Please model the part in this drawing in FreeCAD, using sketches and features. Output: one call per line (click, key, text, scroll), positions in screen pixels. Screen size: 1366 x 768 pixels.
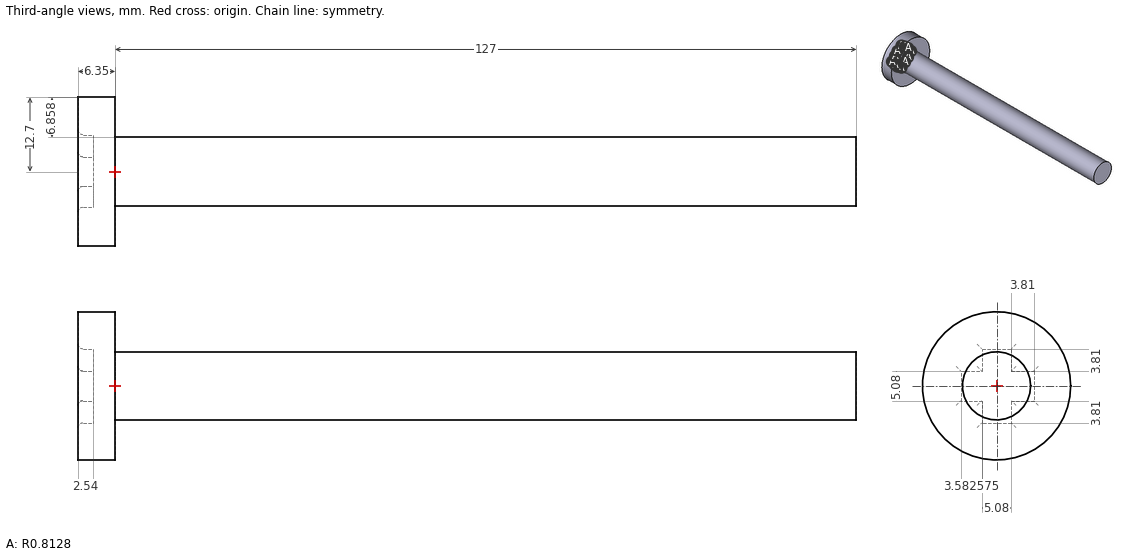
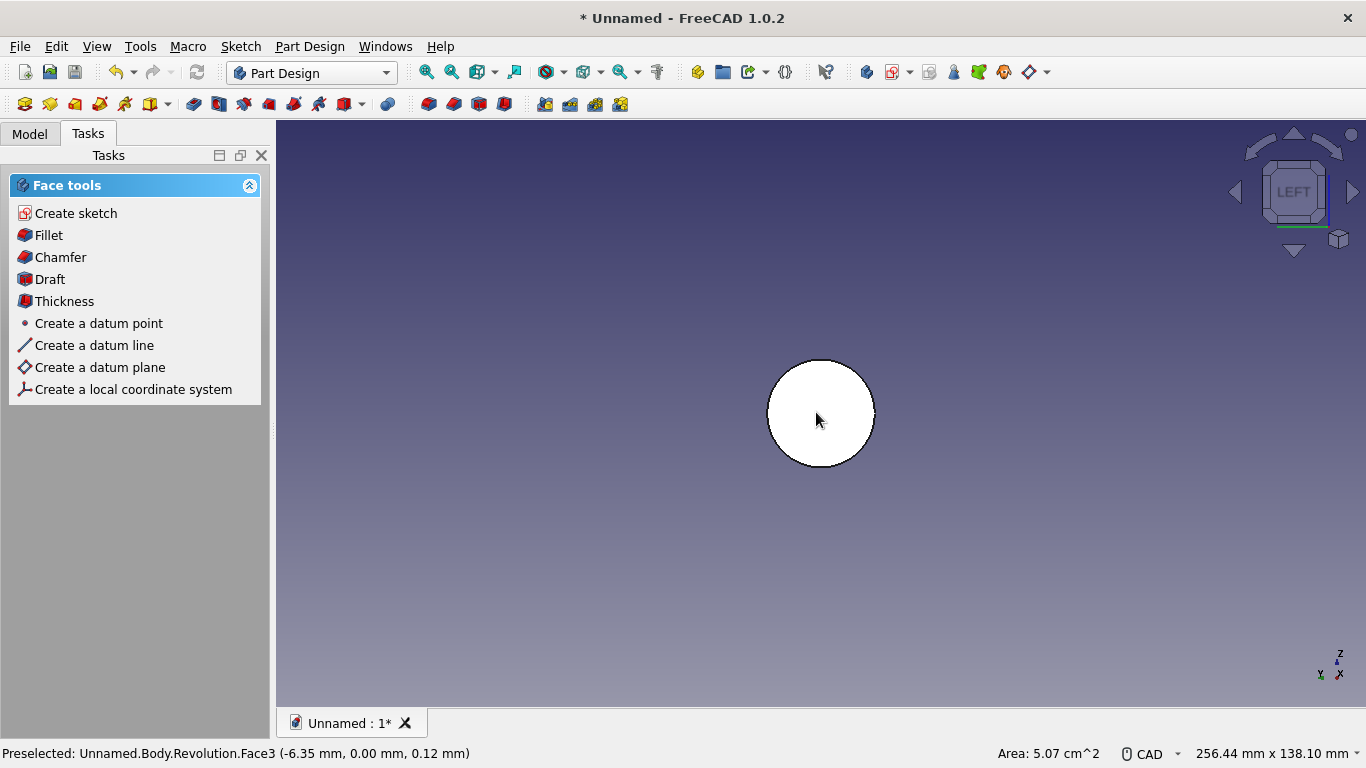
click(892, 72)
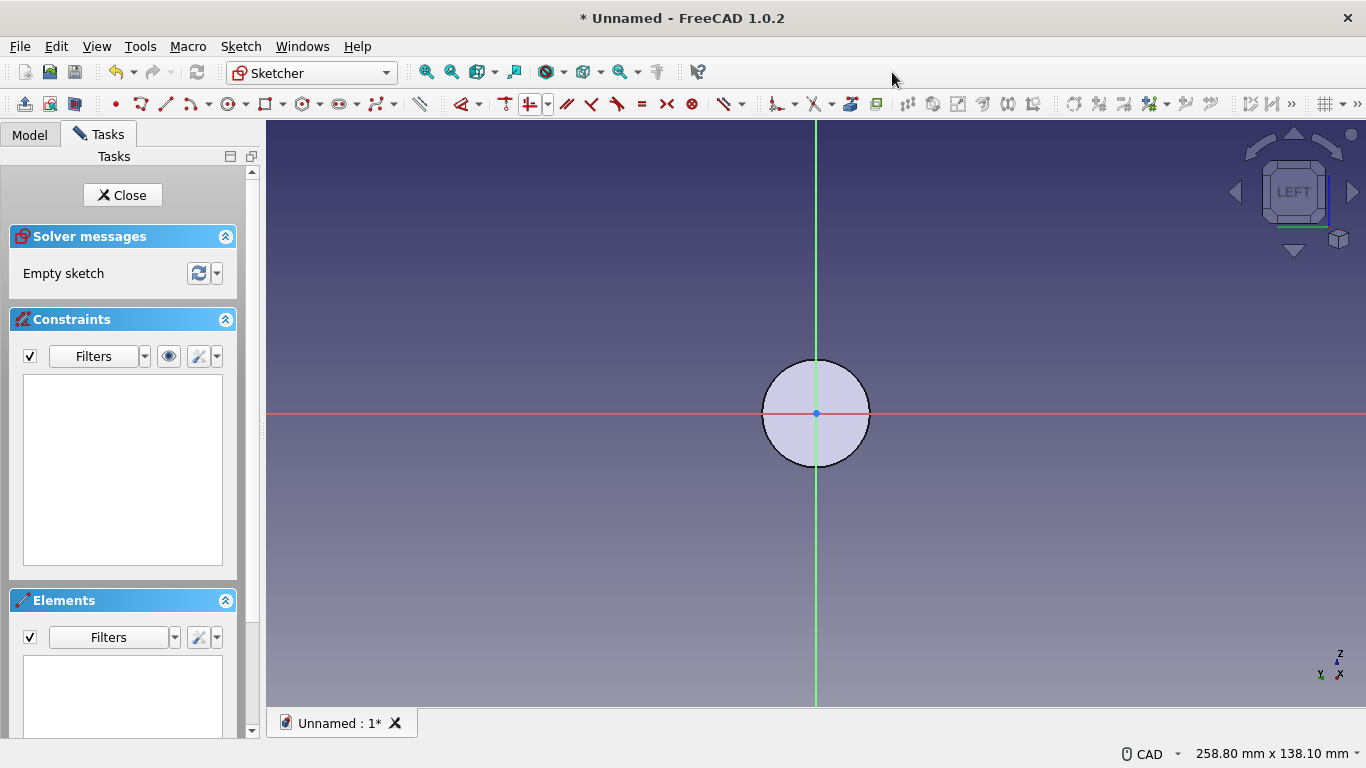
scroll(826, 414, up, 10)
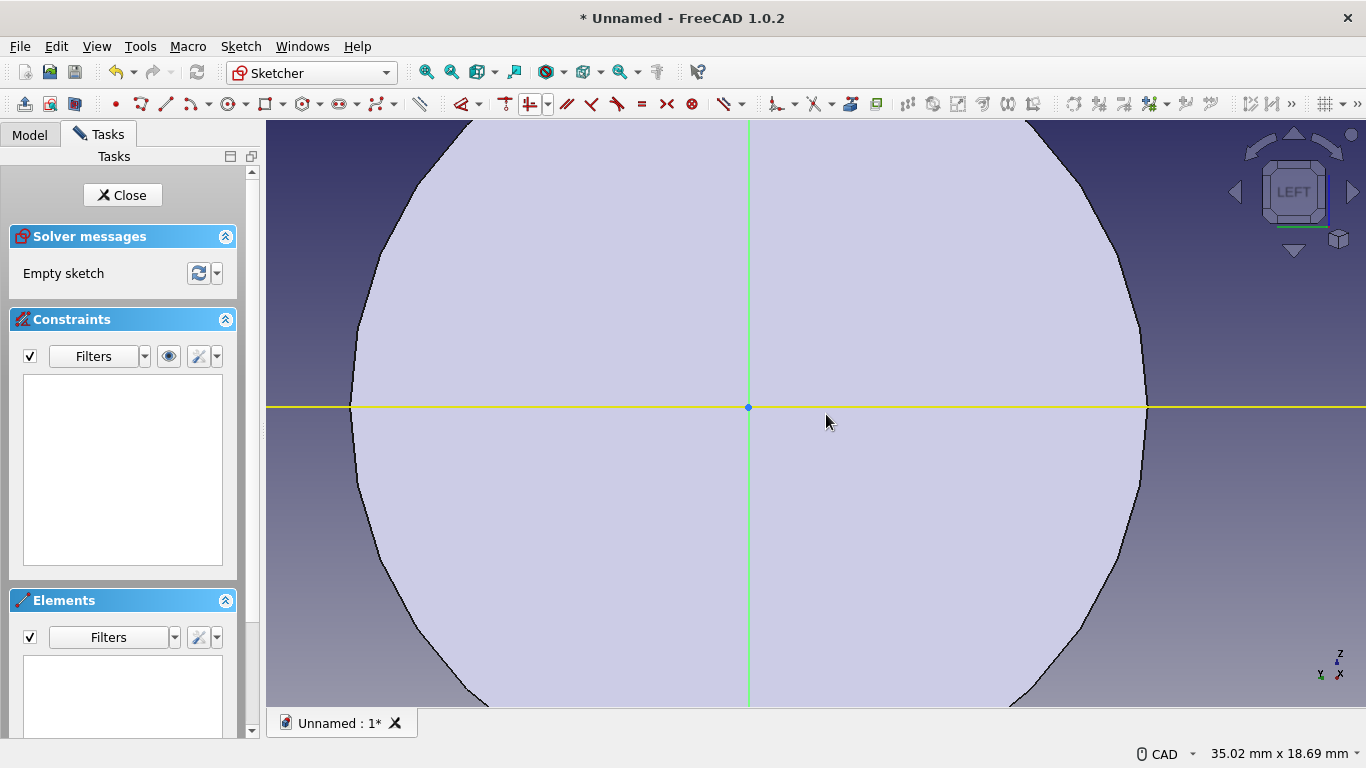
click(141, 104)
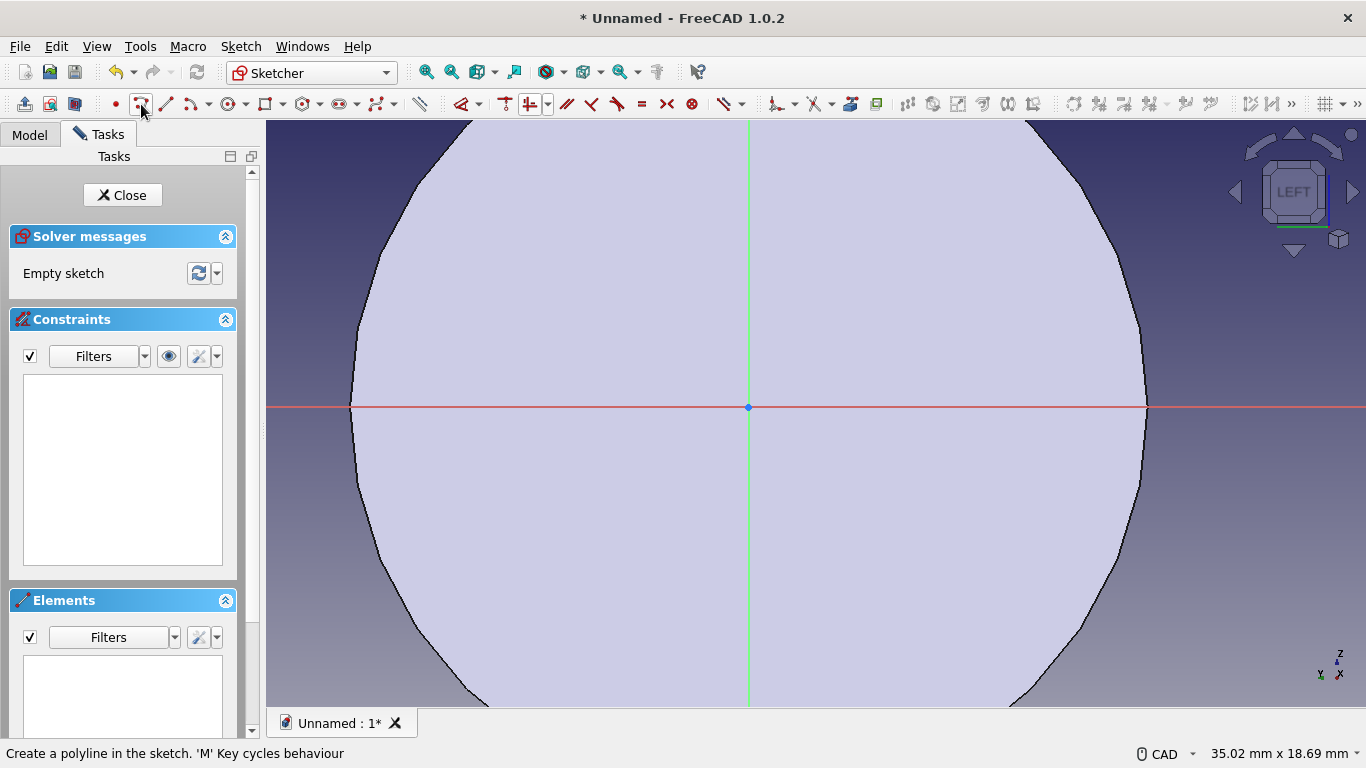
click(669, 487)
click(669, 607)
click(829, 607)
click(829, 487)
click(941, 487)
click(941, 327)
click(829, 327)
click(829, 208)
click(669, 208)
click(669, 327)
click(549, 327)
click(549, 487)
click(669, 488)
key(Escape)
key(Escape)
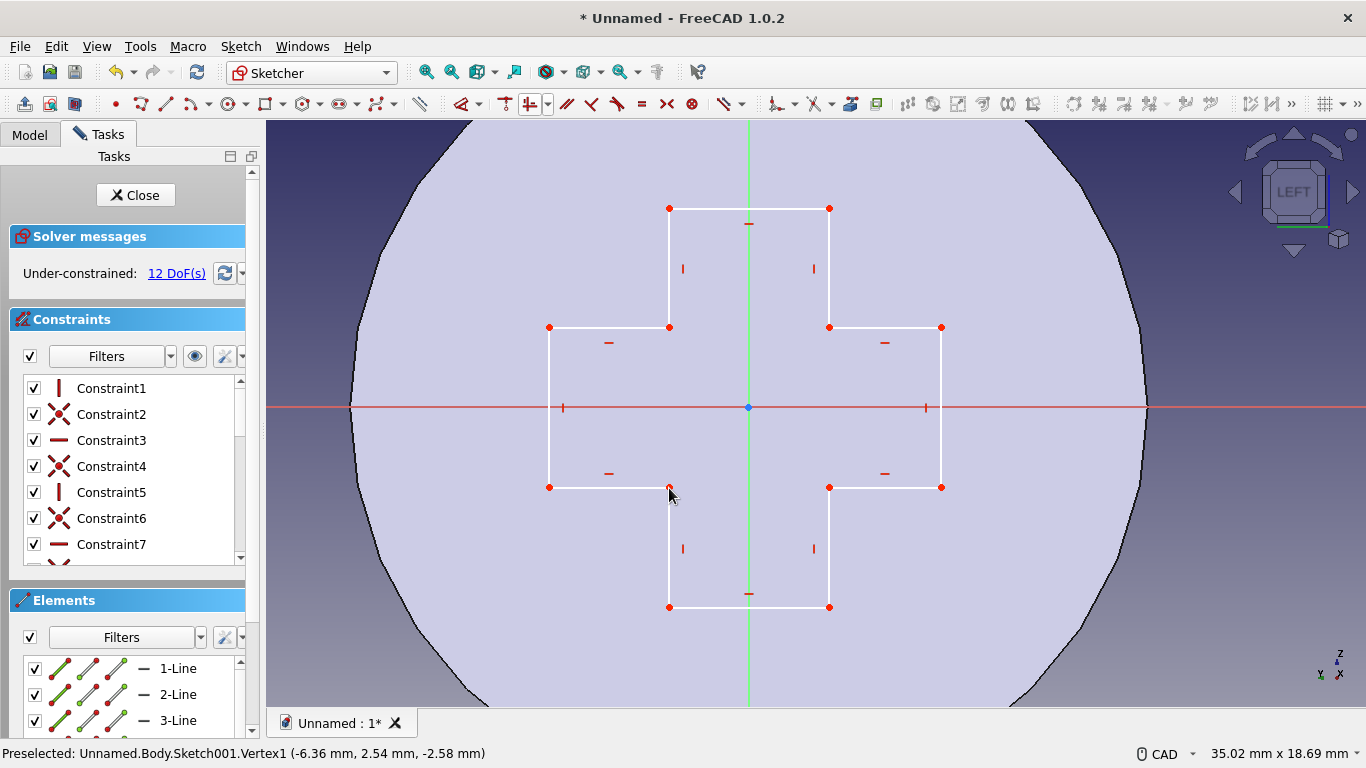
click(669, 488)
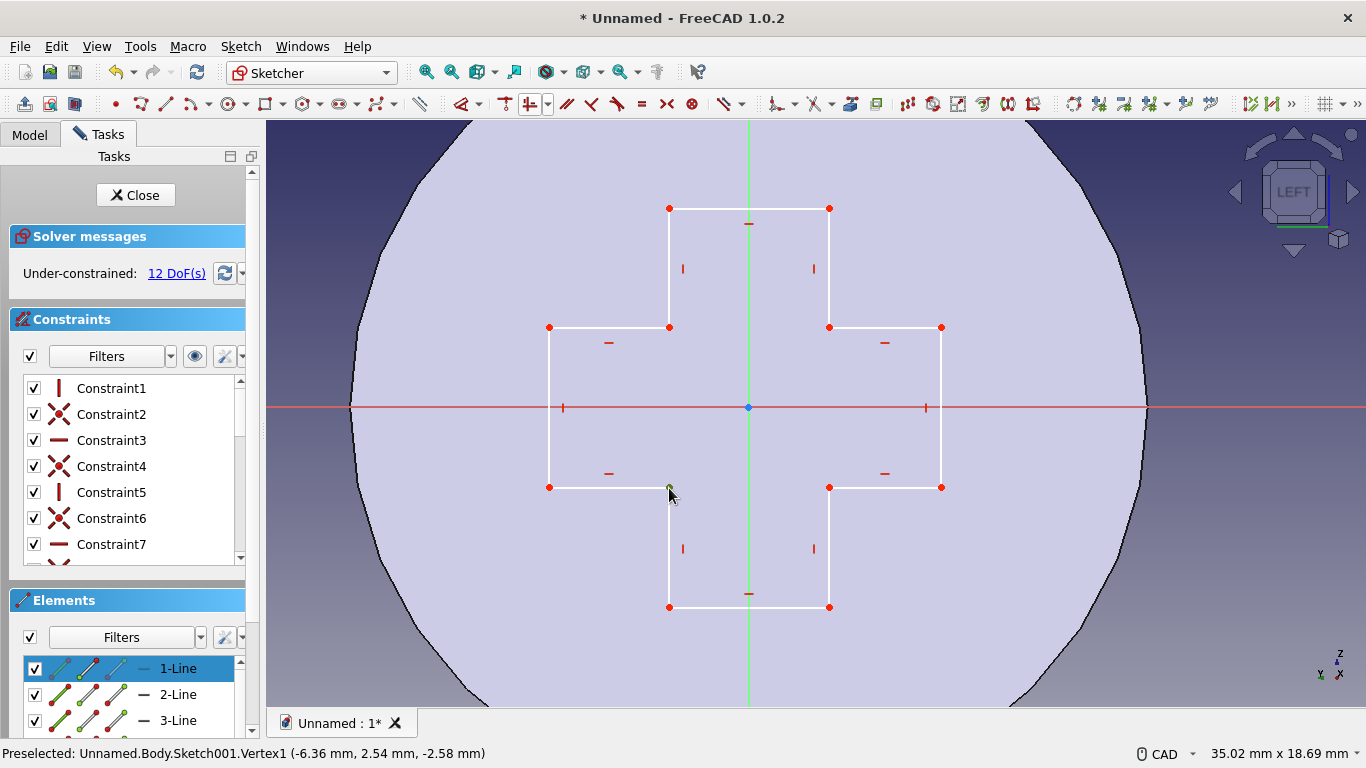
click(829, 488)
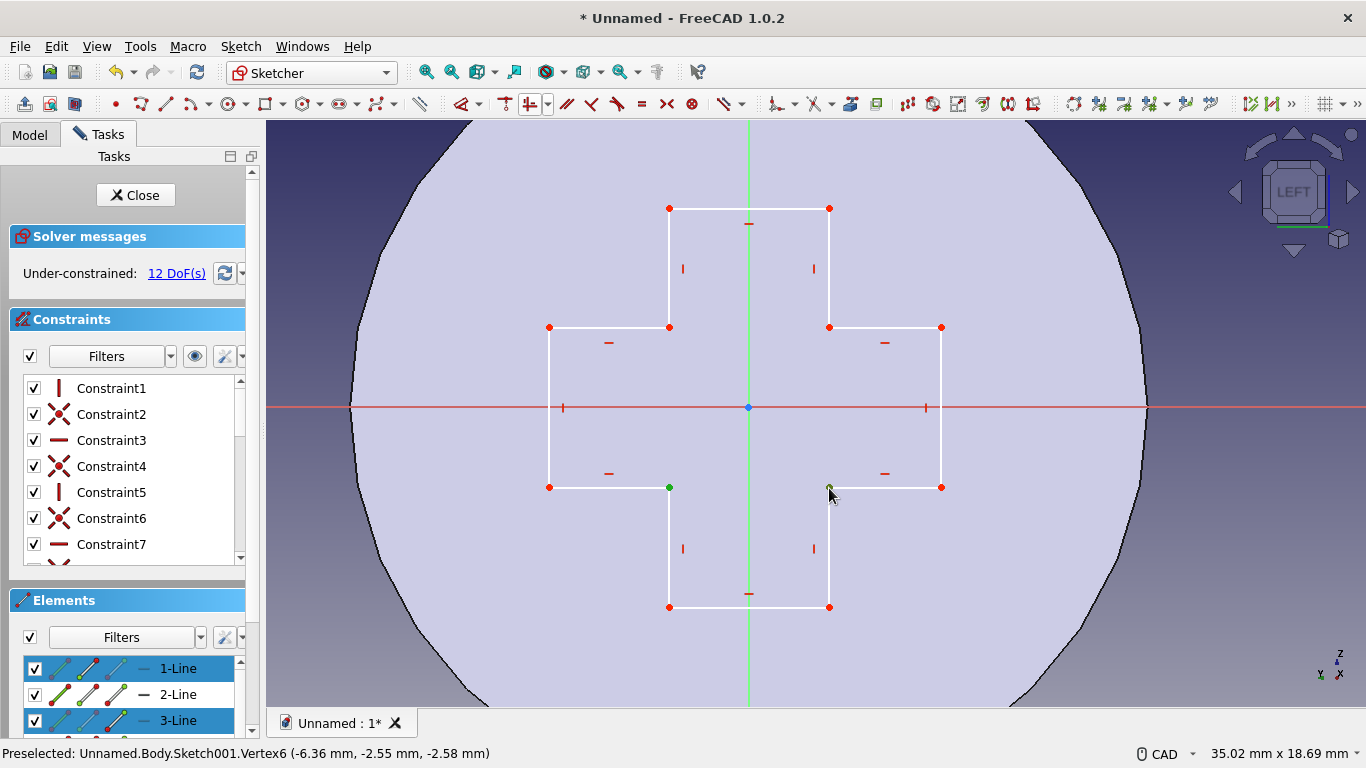
click(749, 641)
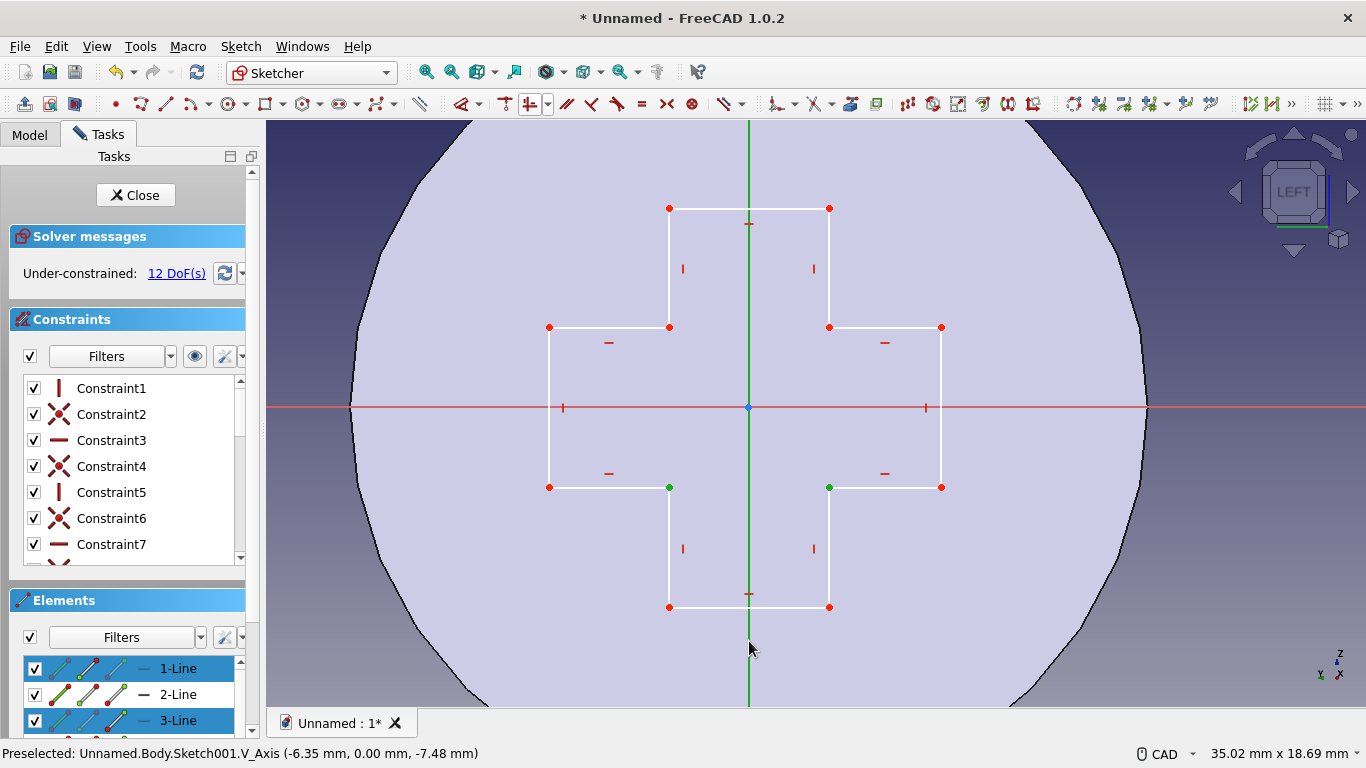
click(667, 104)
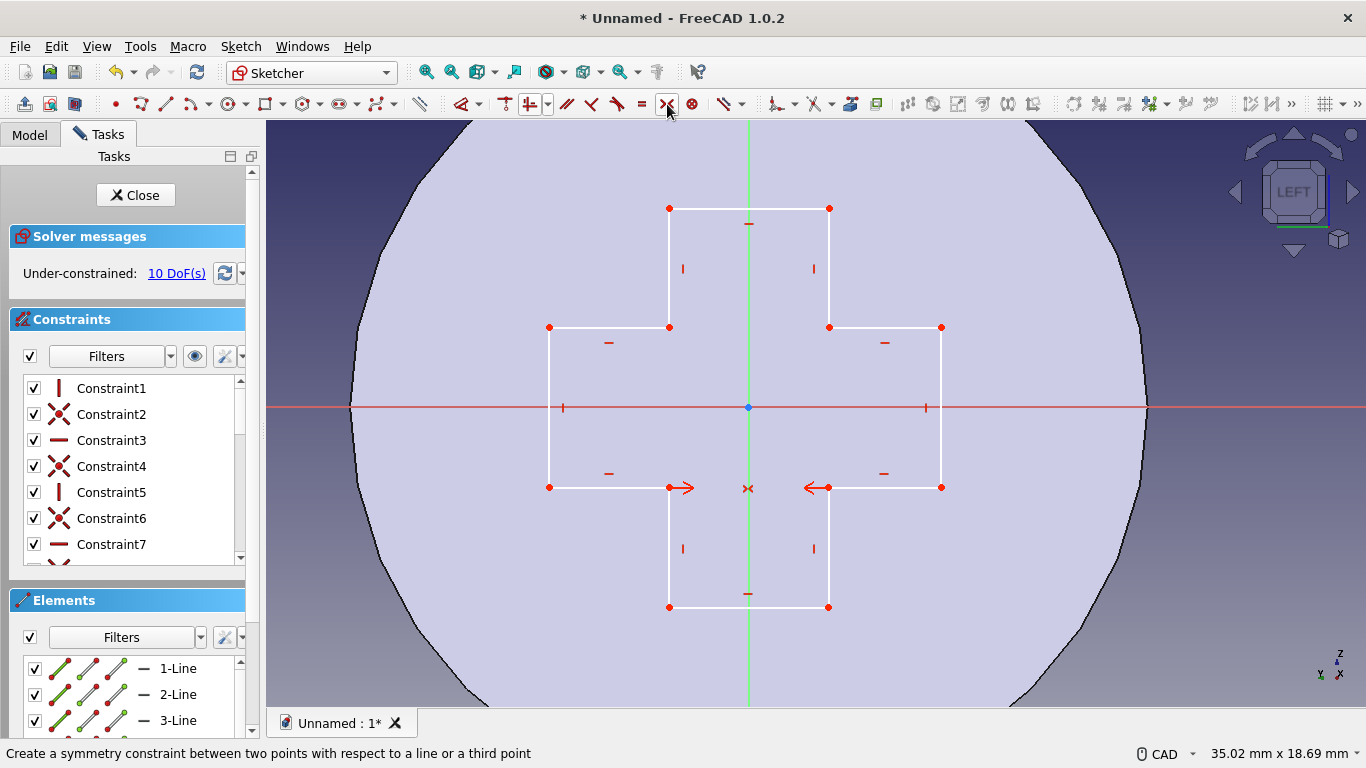
click(829, 488)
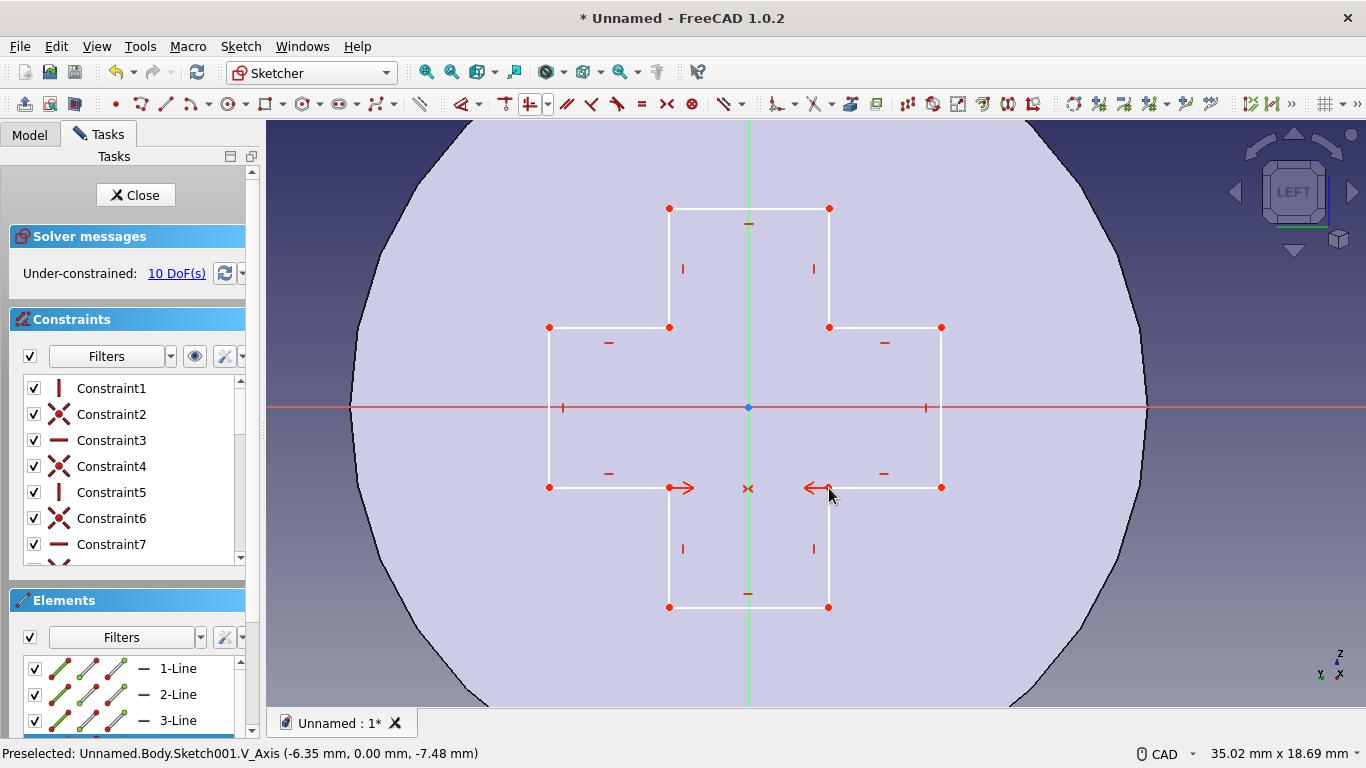
click(829, 328)